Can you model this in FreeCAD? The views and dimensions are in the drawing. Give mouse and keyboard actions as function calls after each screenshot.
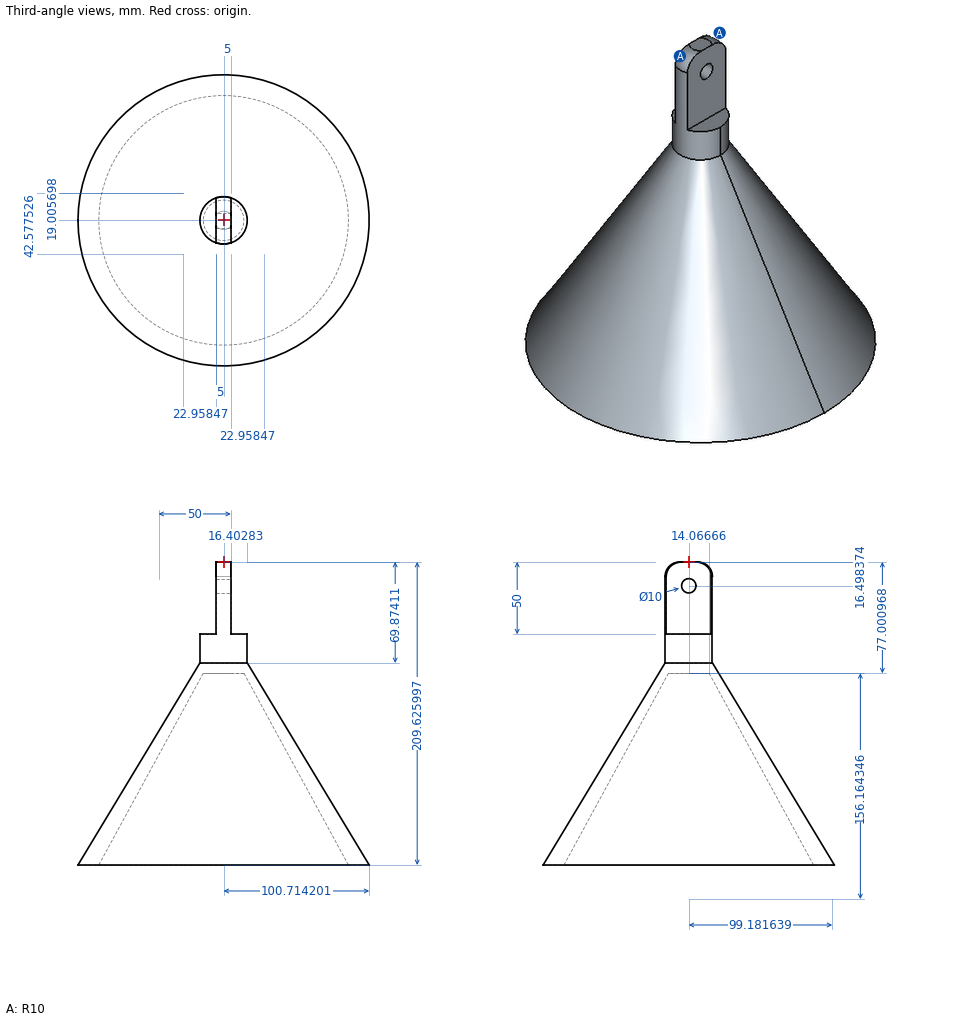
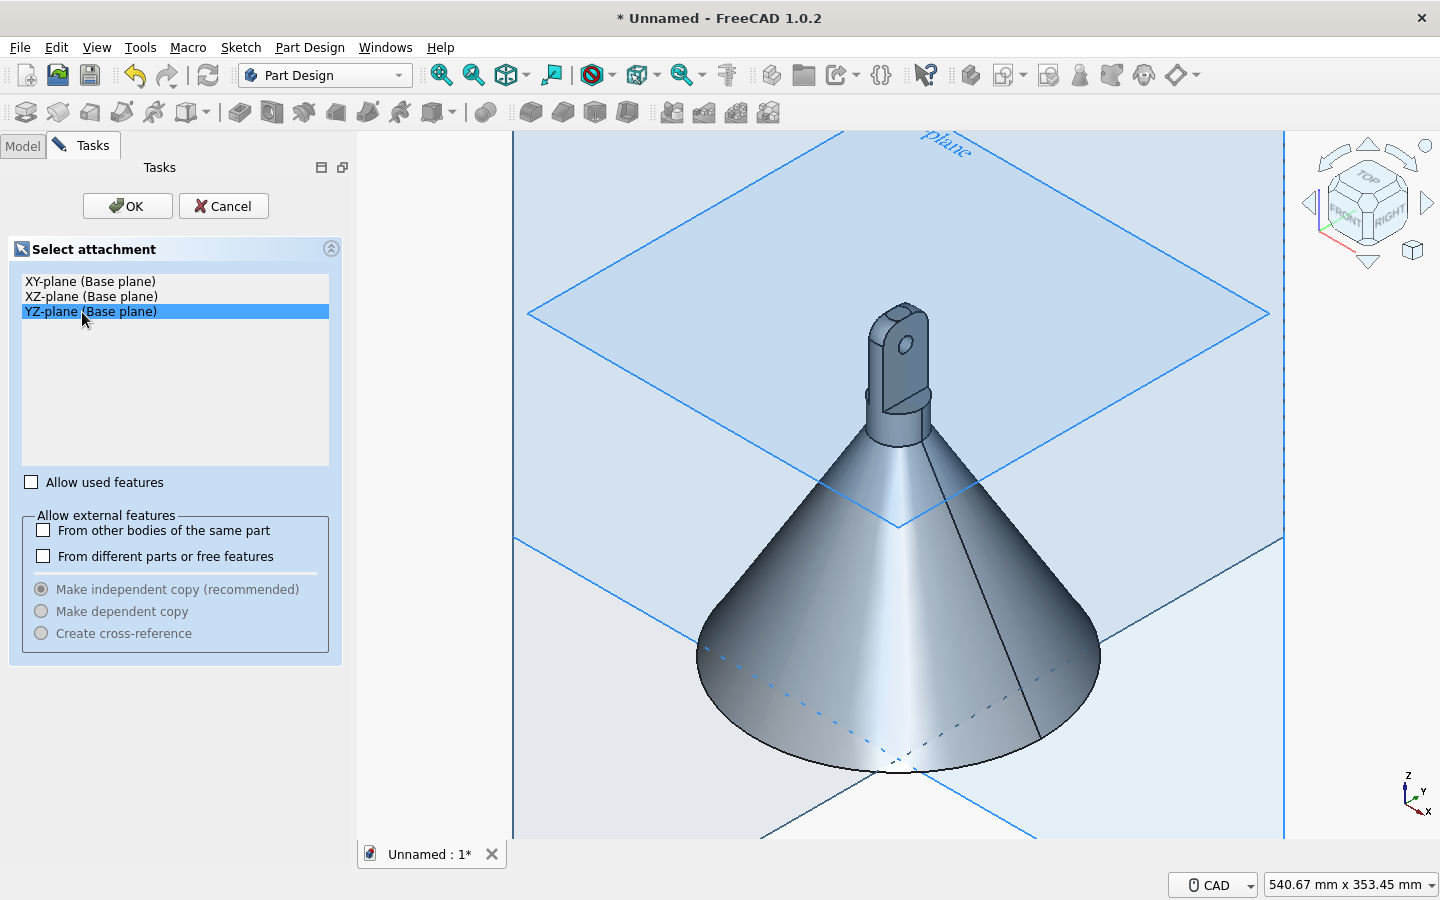
click(128, 206)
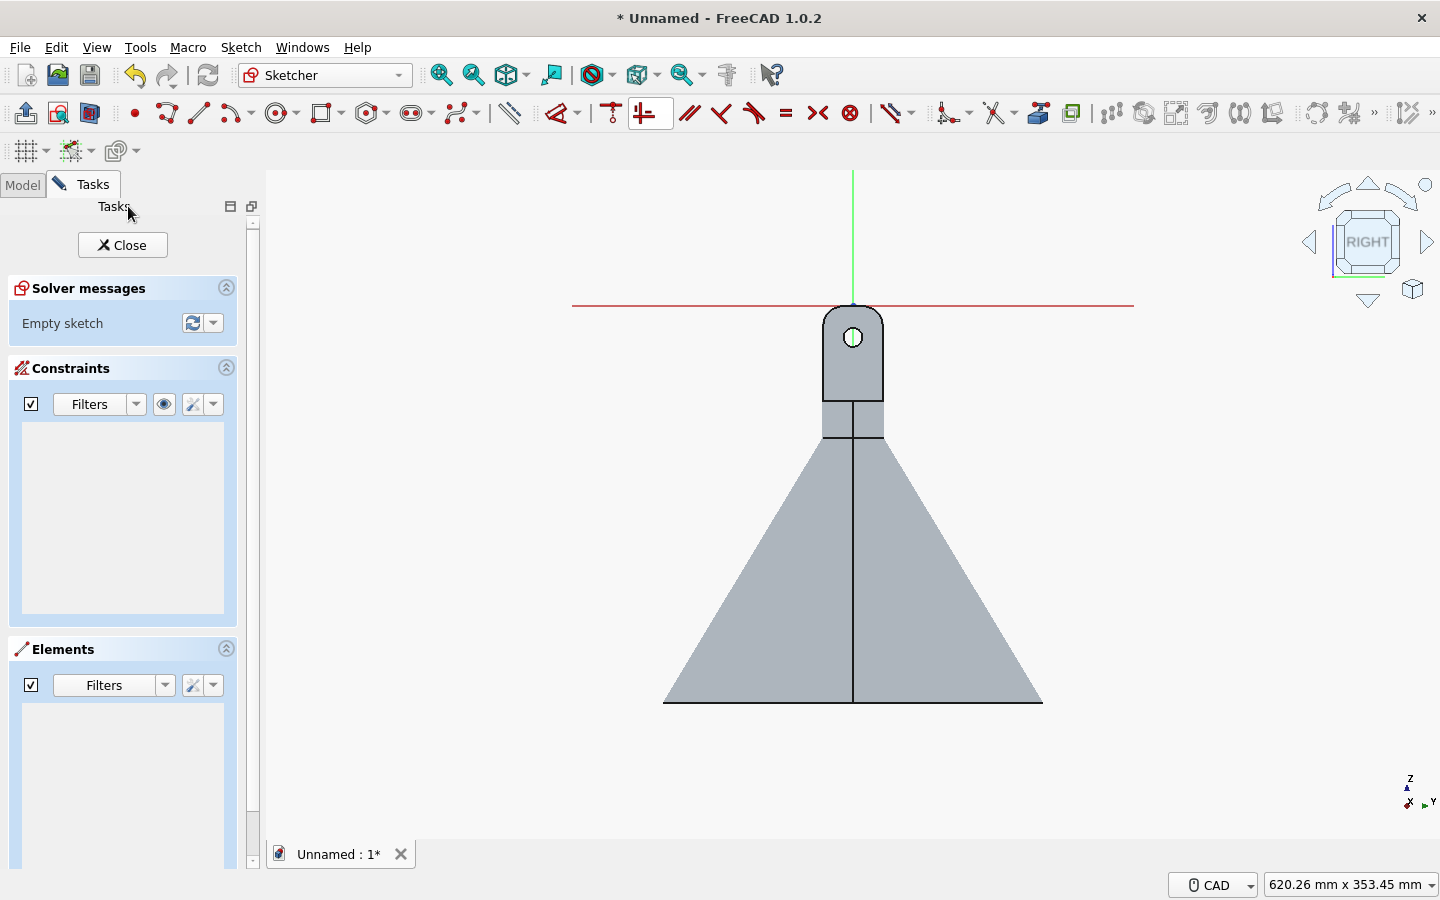
click(90, 114)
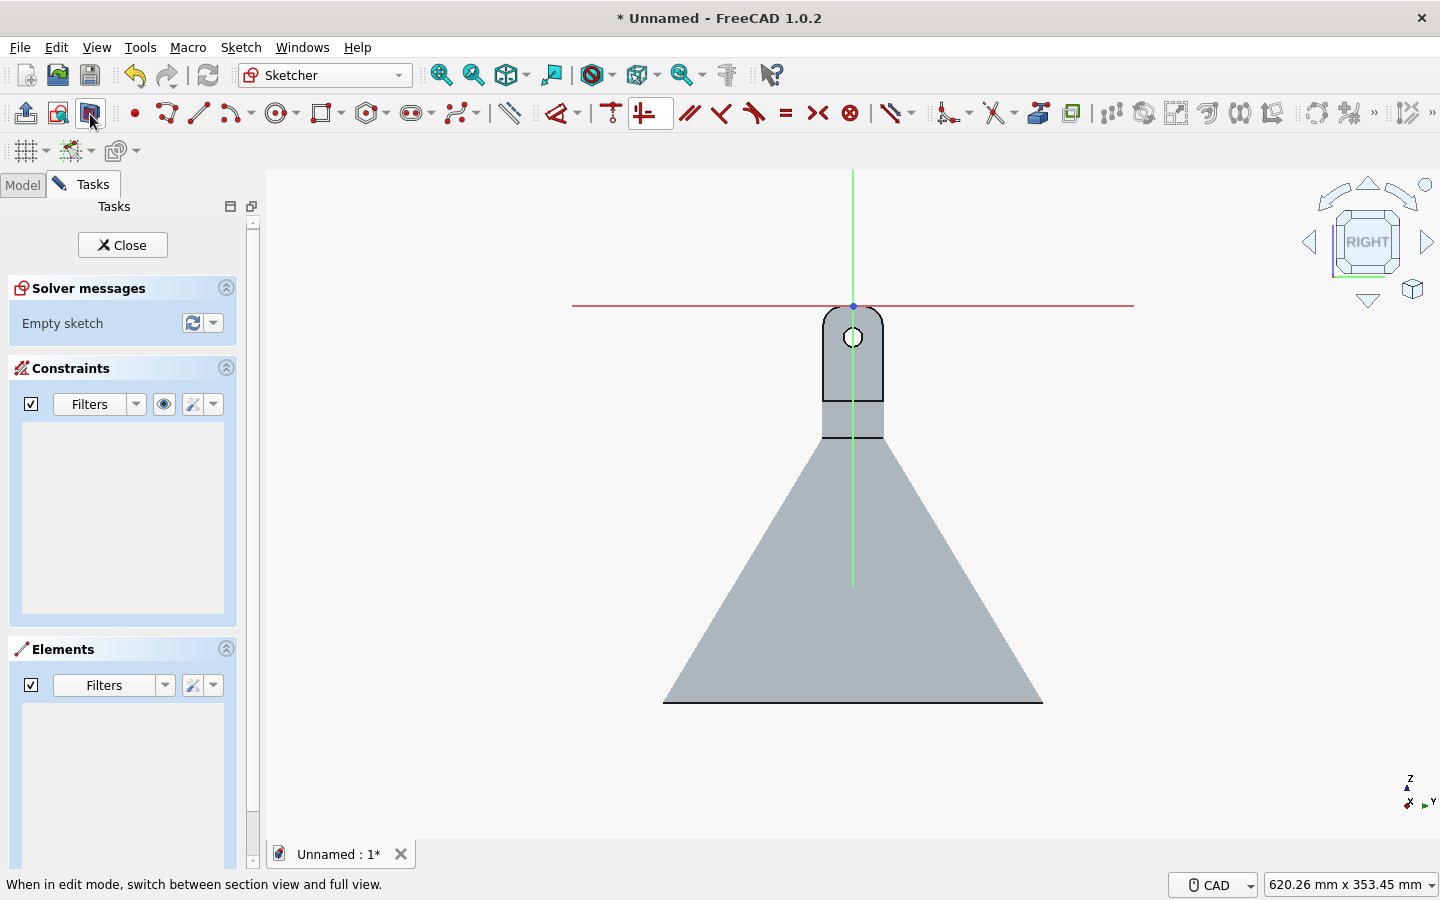
click(168, 114)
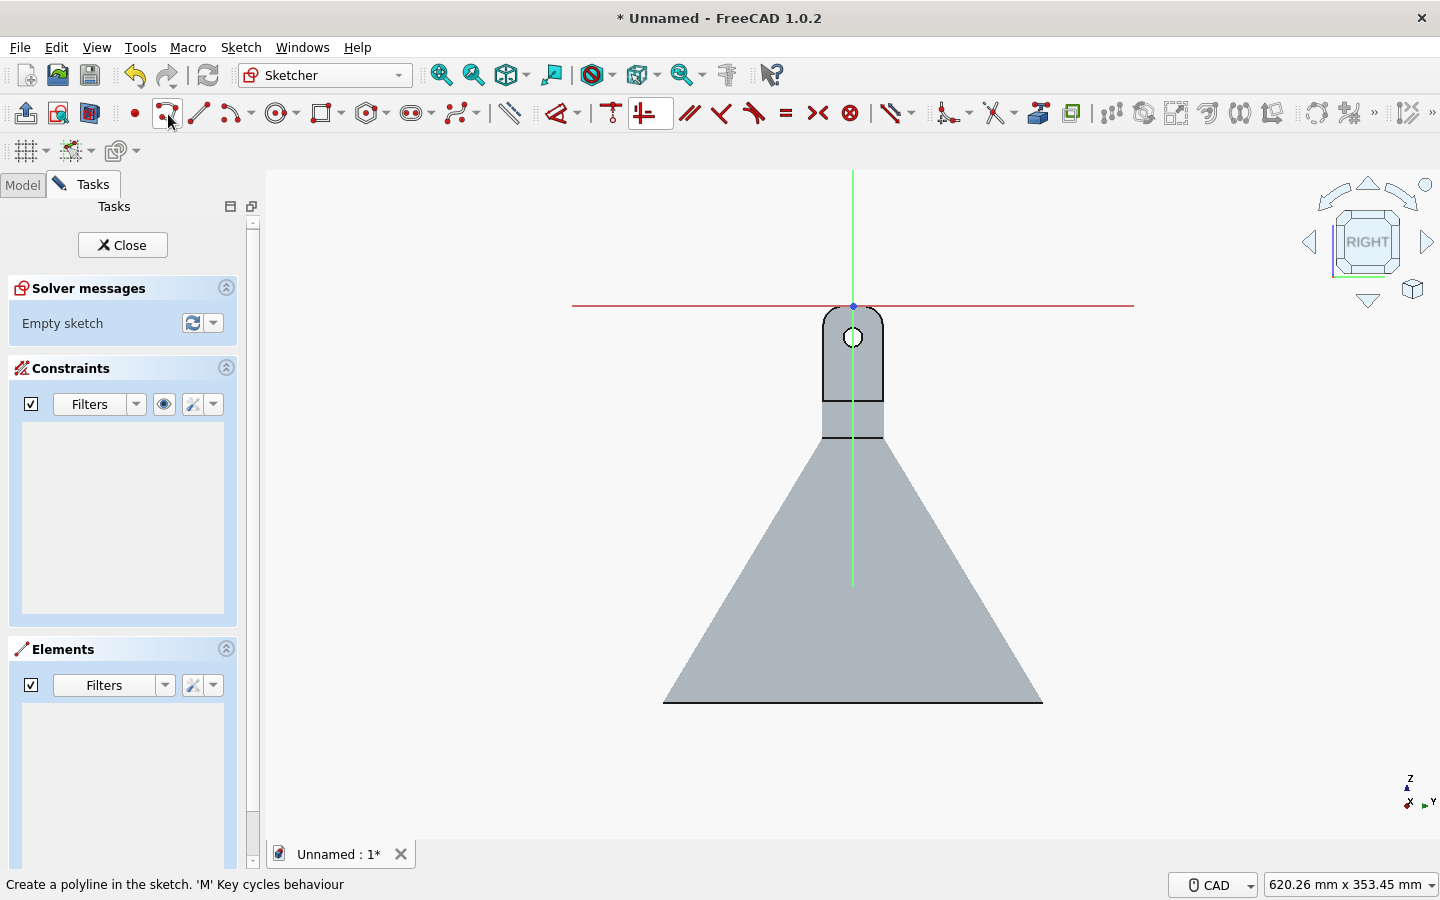
click(853, 452)
click(862, 747)
click(1041, 747)
click(880, 452)
click(853, 453)
key(Escape)
key(Escape)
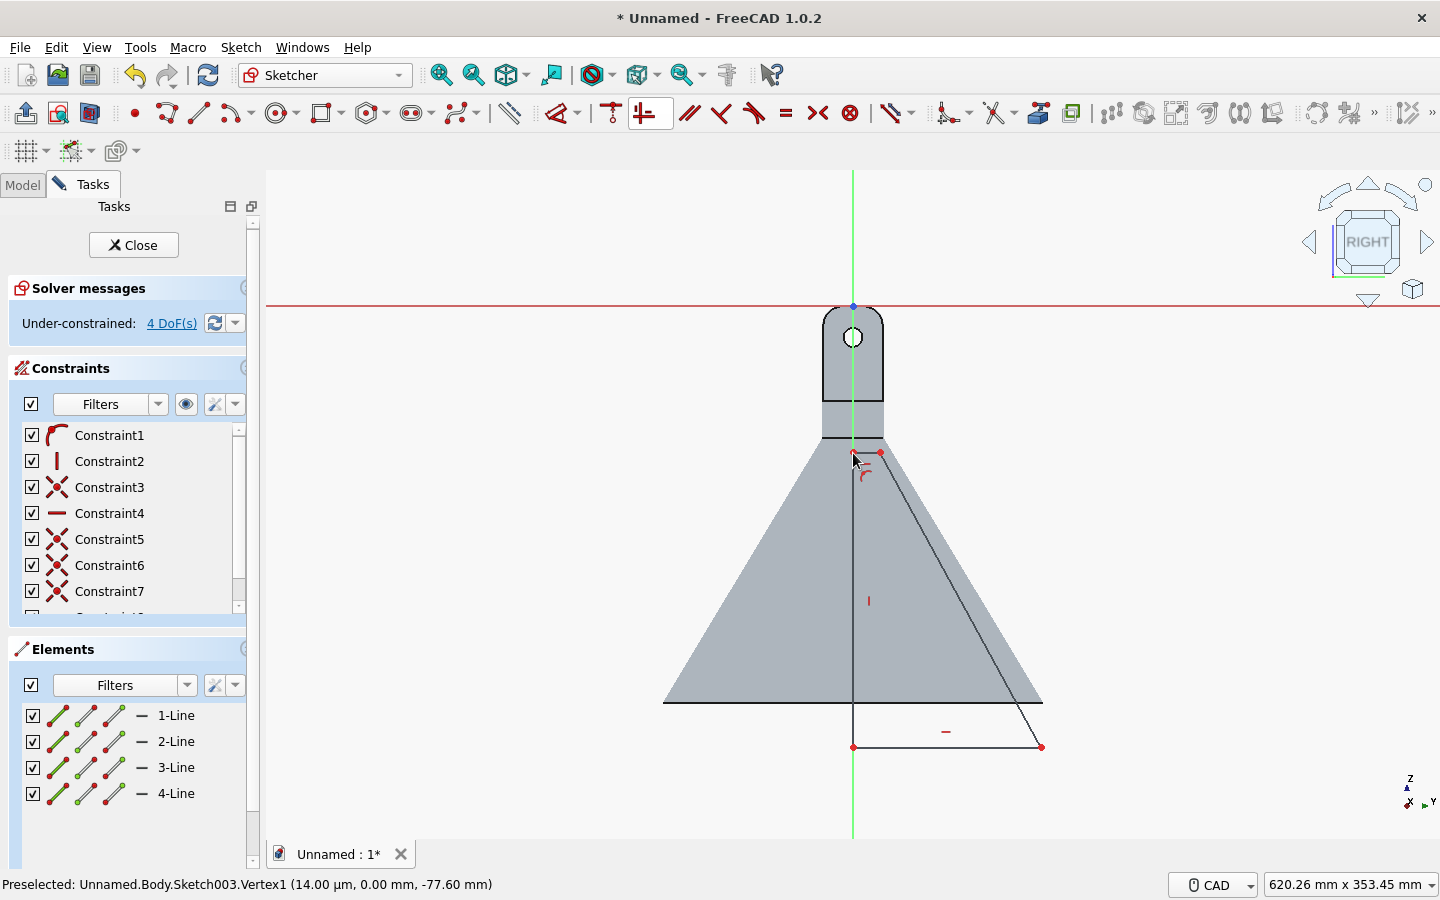
click(556, 114)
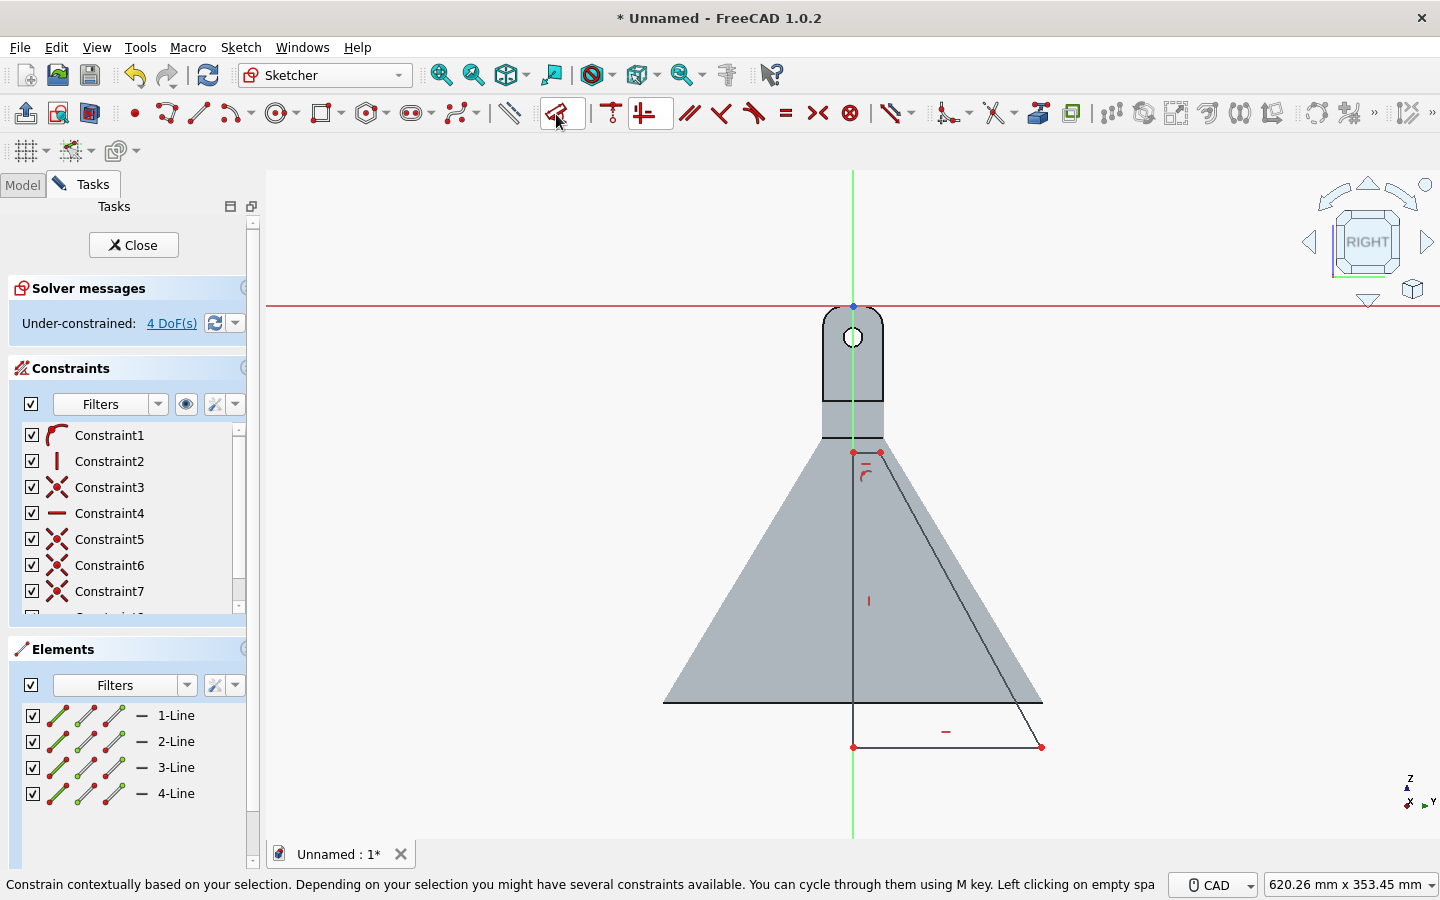
scroll(869, 453, up, 2)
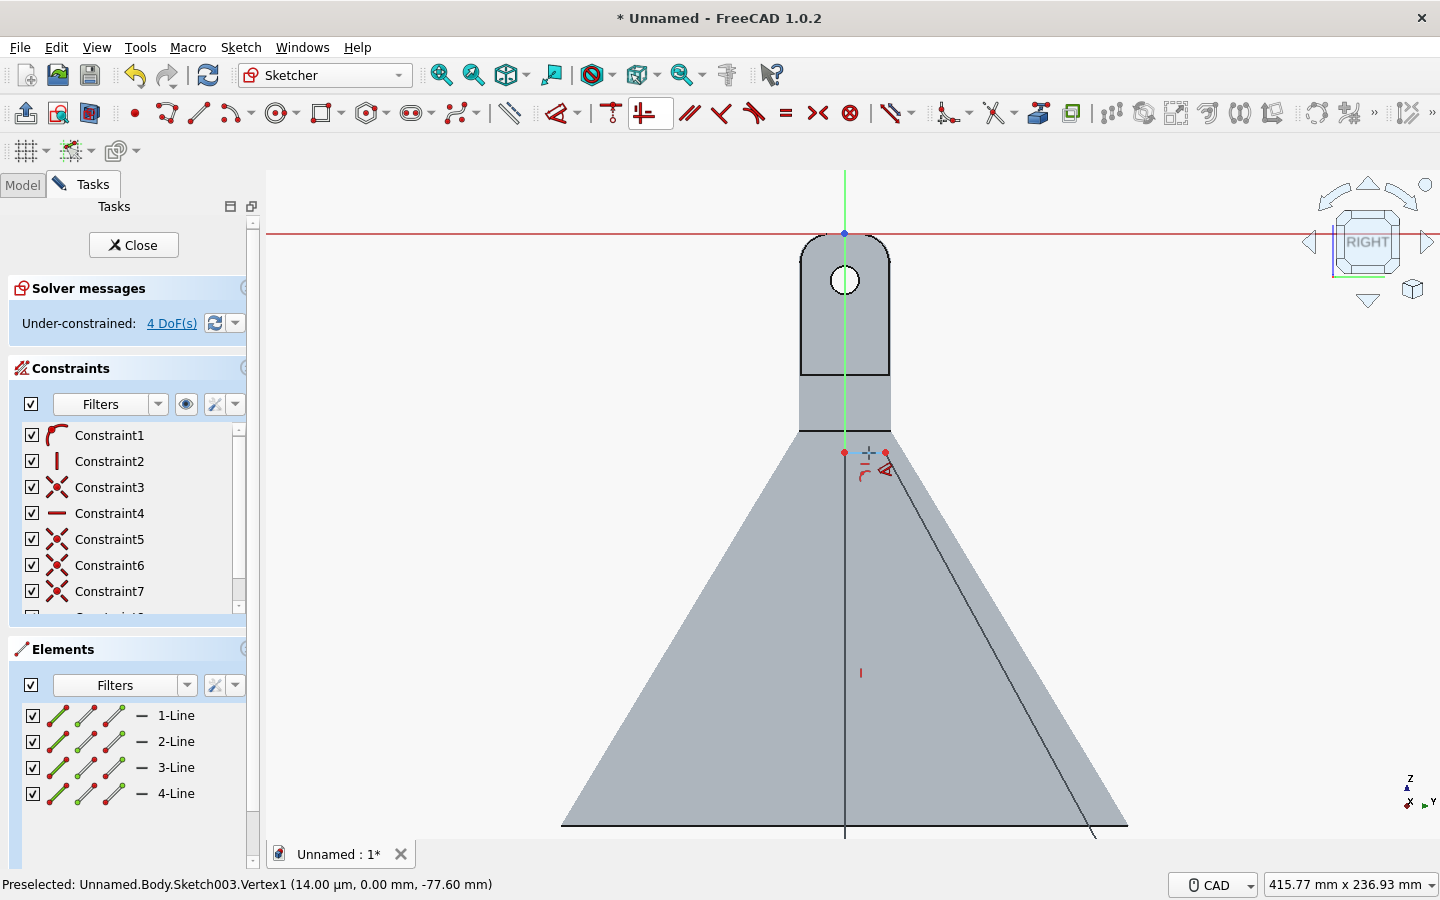
click(869, 453)
click(865, 419)